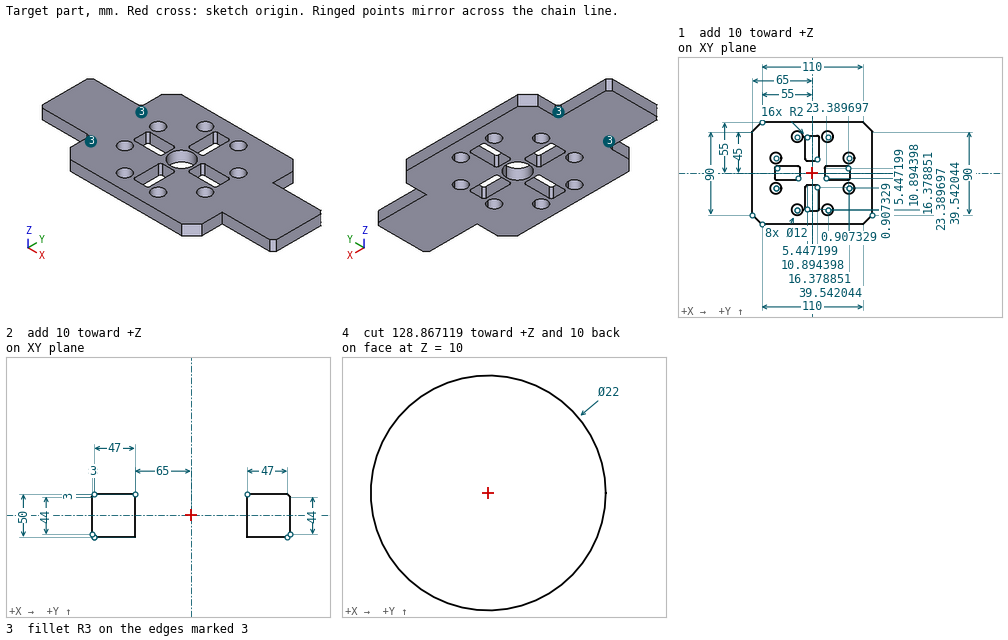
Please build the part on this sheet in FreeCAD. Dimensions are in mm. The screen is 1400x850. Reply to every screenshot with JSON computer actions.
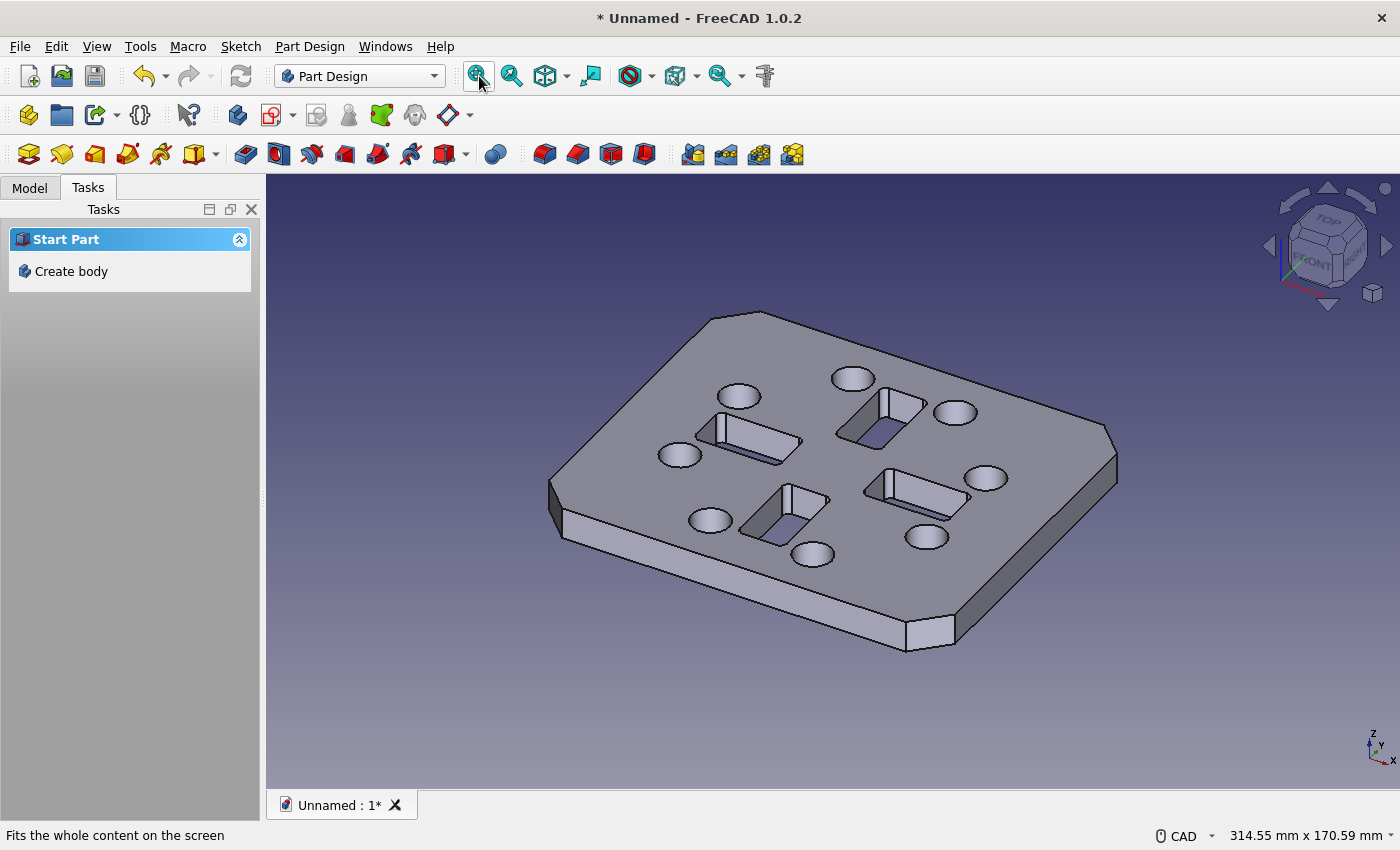
{"action": "left_click", "coordinate": [270, 116]}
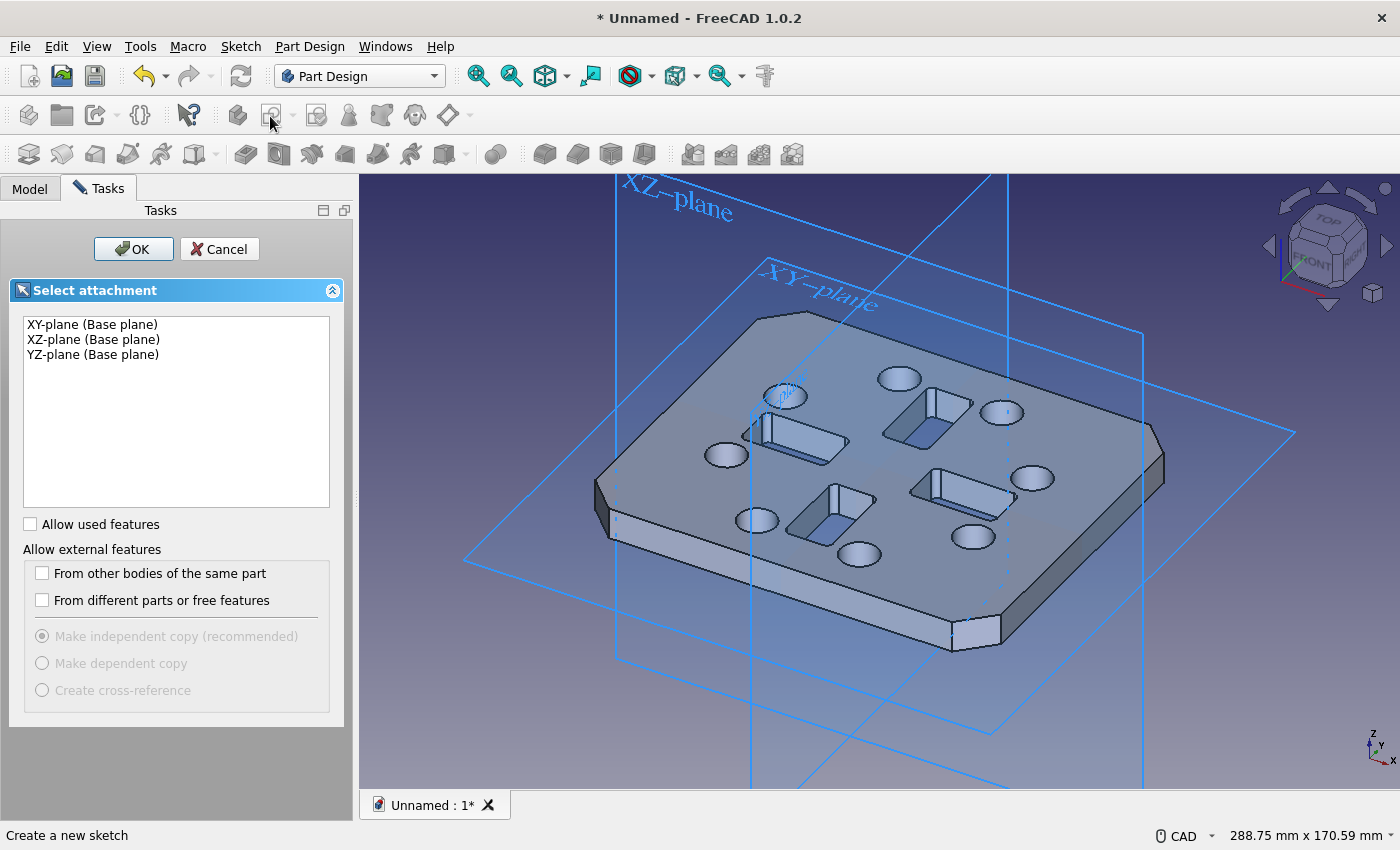
{"action": "left_click", "coordinate": [84, 324]}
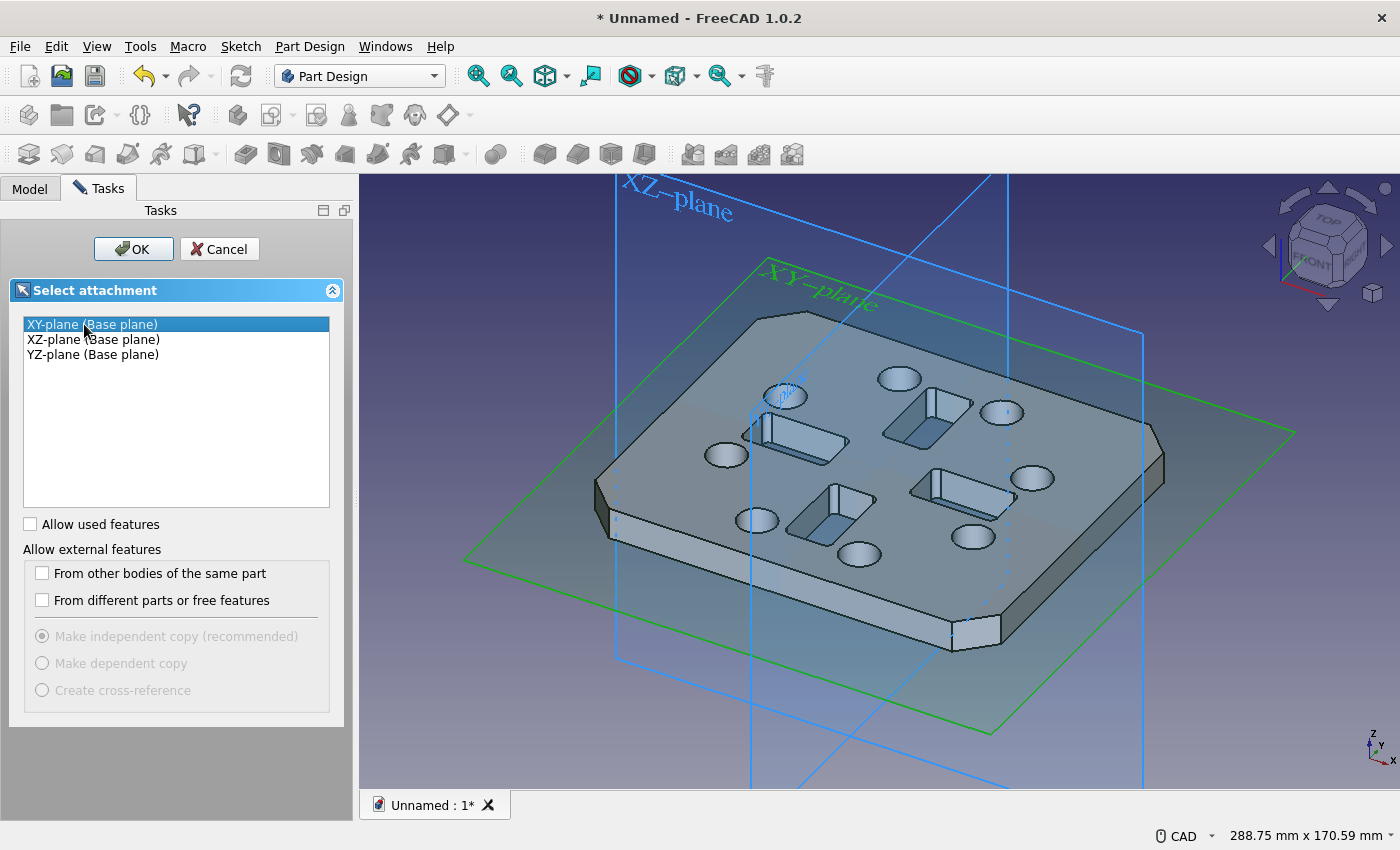
{"action": "left_click", "coordinate": [134, 249]}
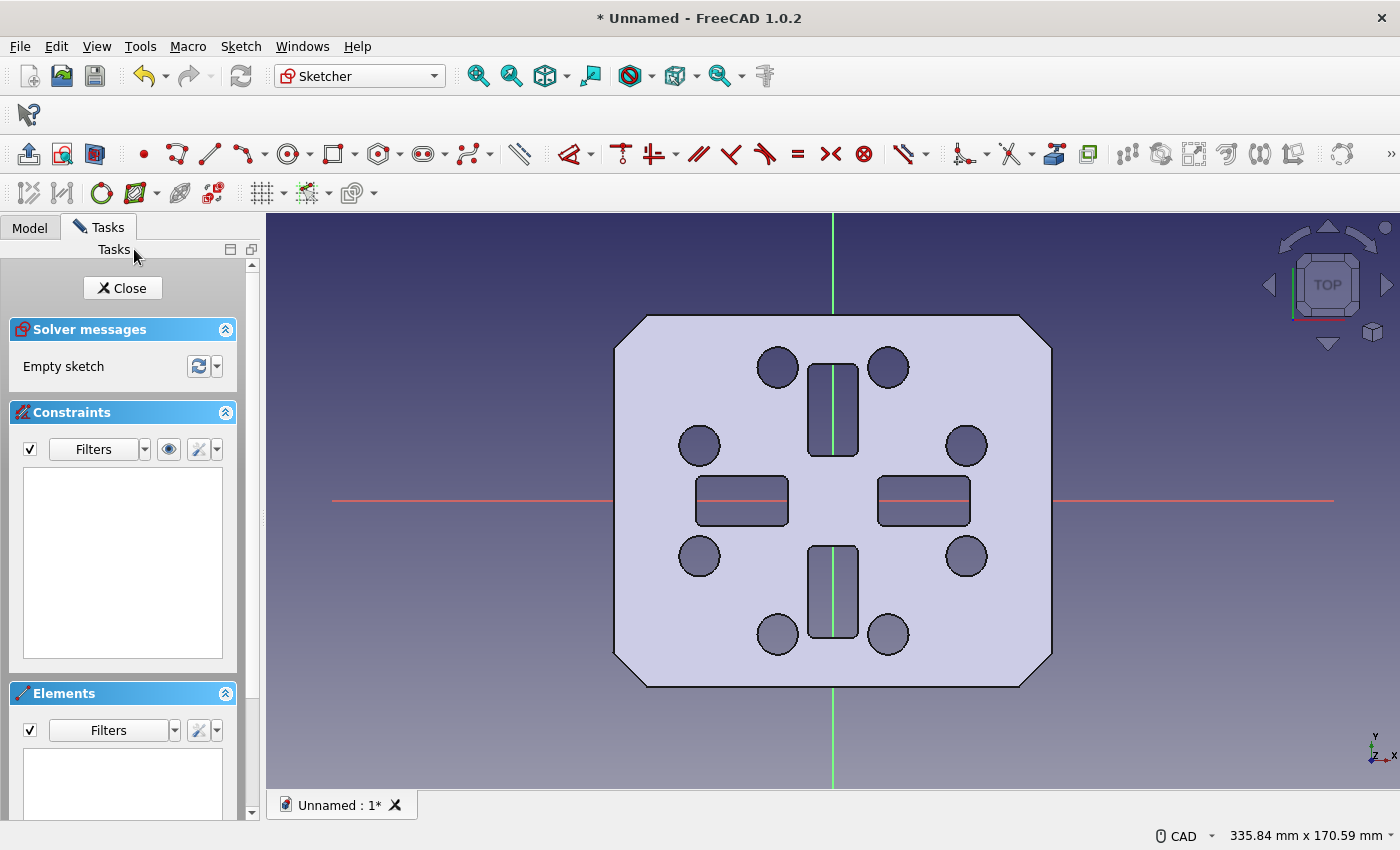
{"action": "left_click", "coordinate": [95, 154]}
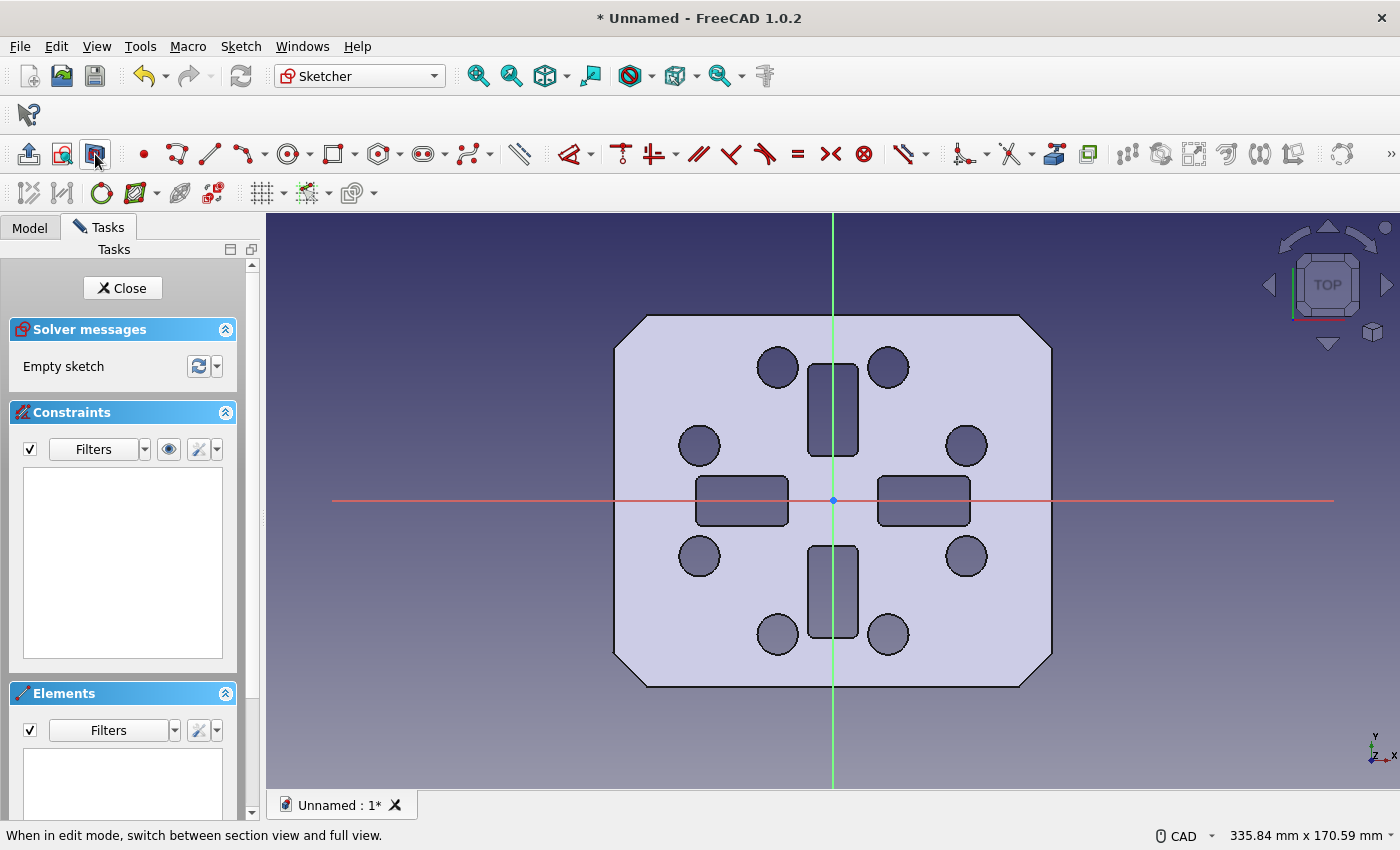
{"action": "scroll", "coordinate": [455, 501], "scroll_direction": "down", "scroll_amount": 1}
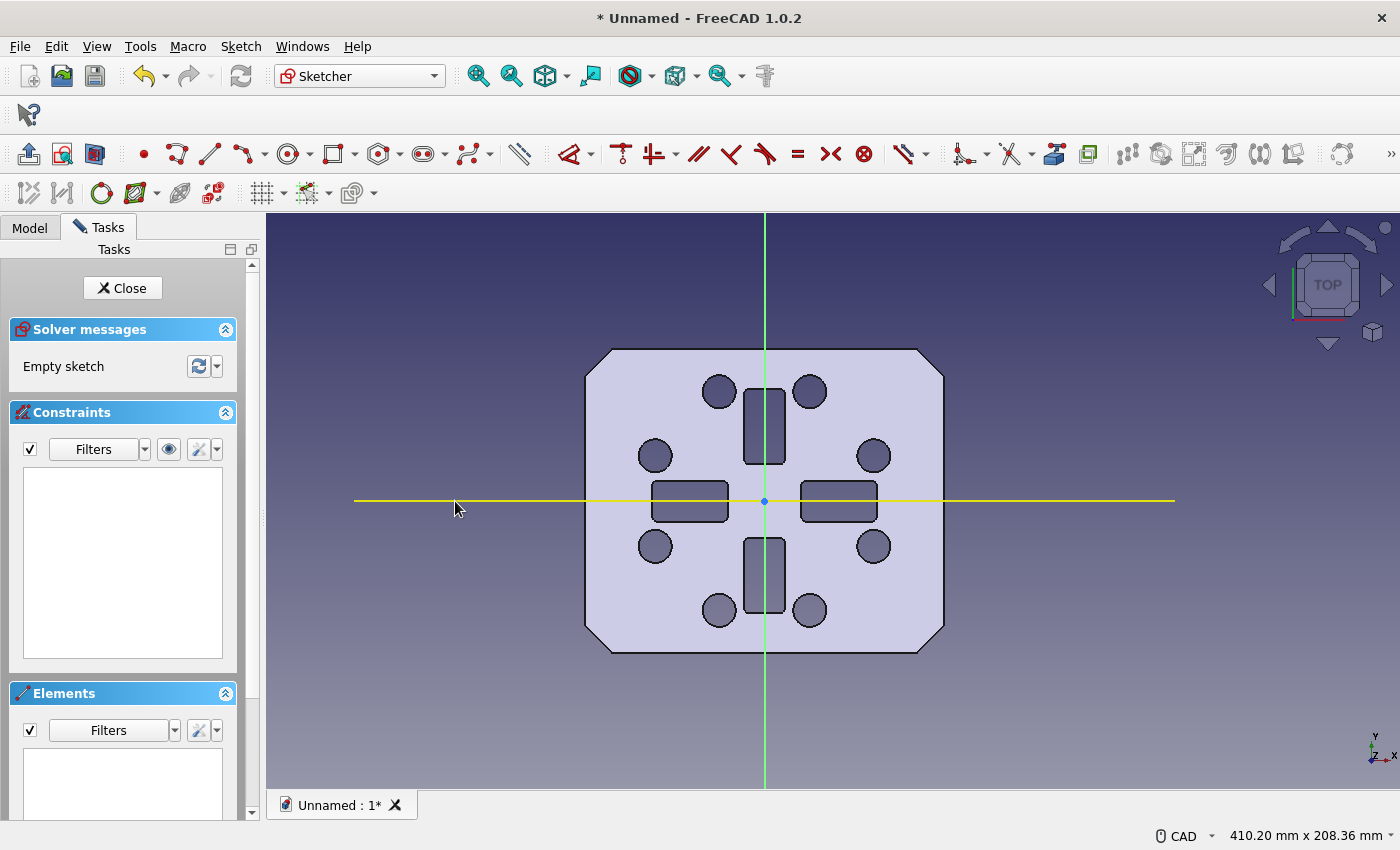
{"action": "left_click", "coordinate": [177, 154]}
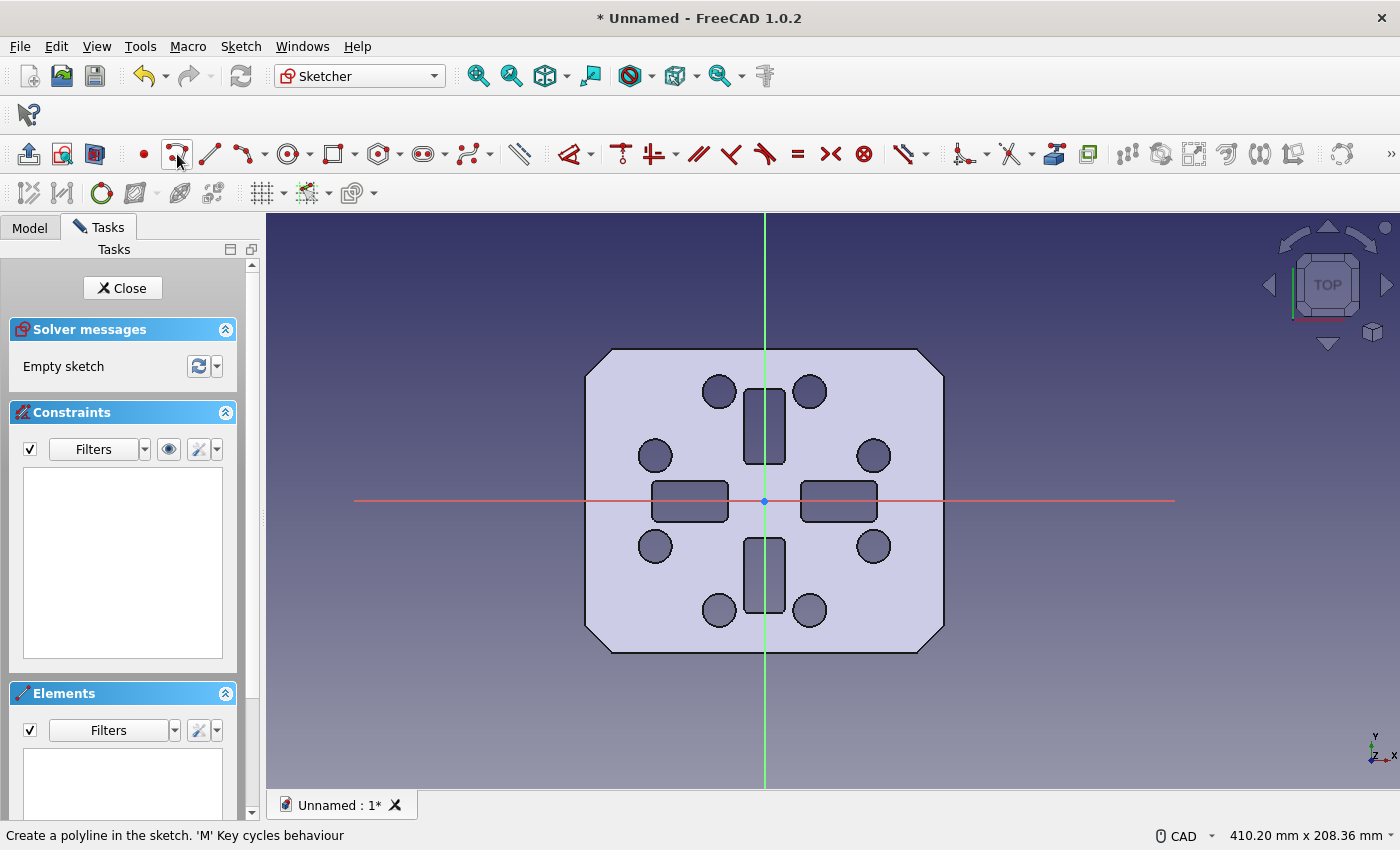
{"action": "left_click", "coordinate": [585, 432]}
{"action": "left_click", "coordinate": [455, 432]}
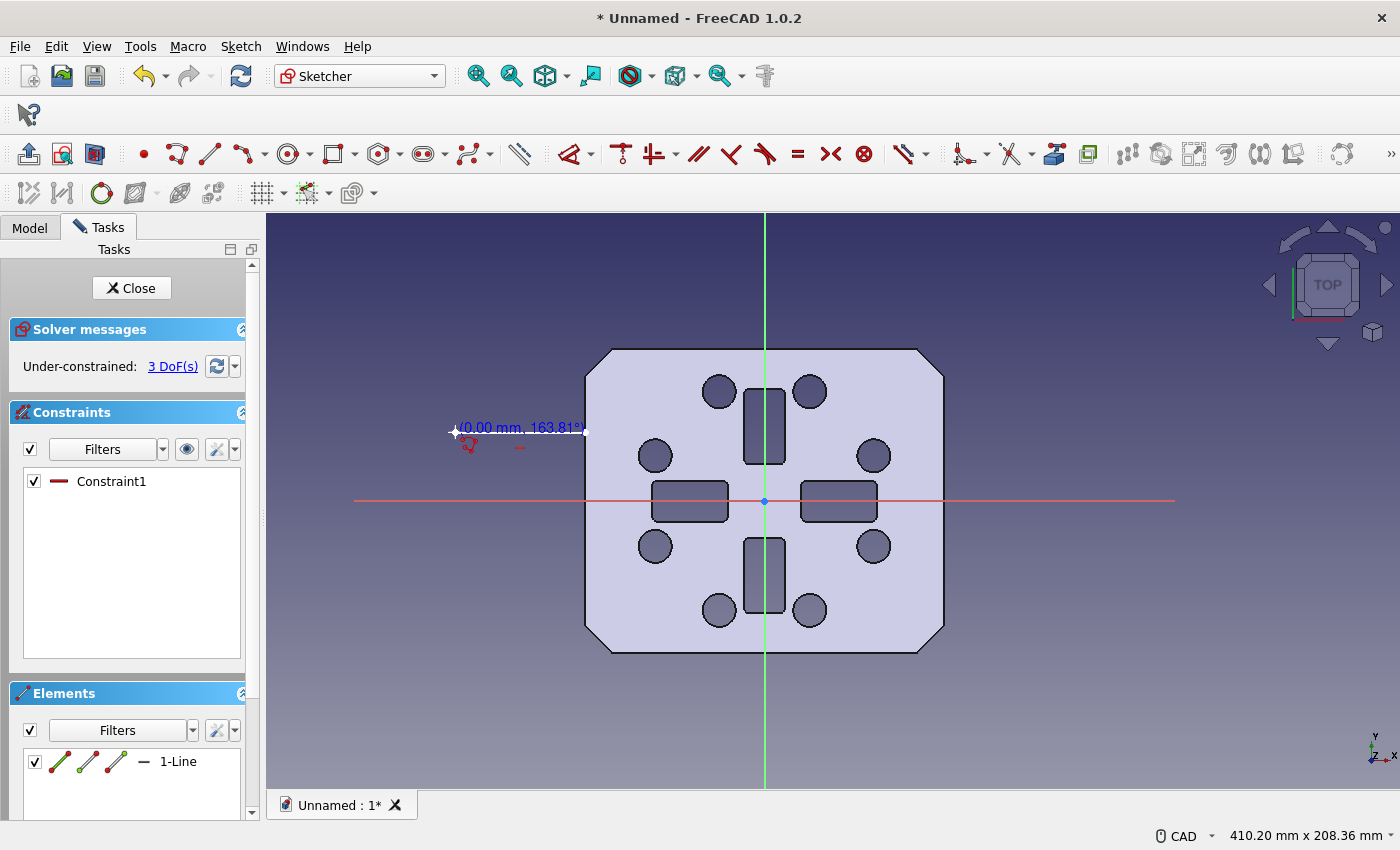
{"action": "scroll", "coordinate": [447, 440], "scroll_direction": "up", "scroll_amount": 2}